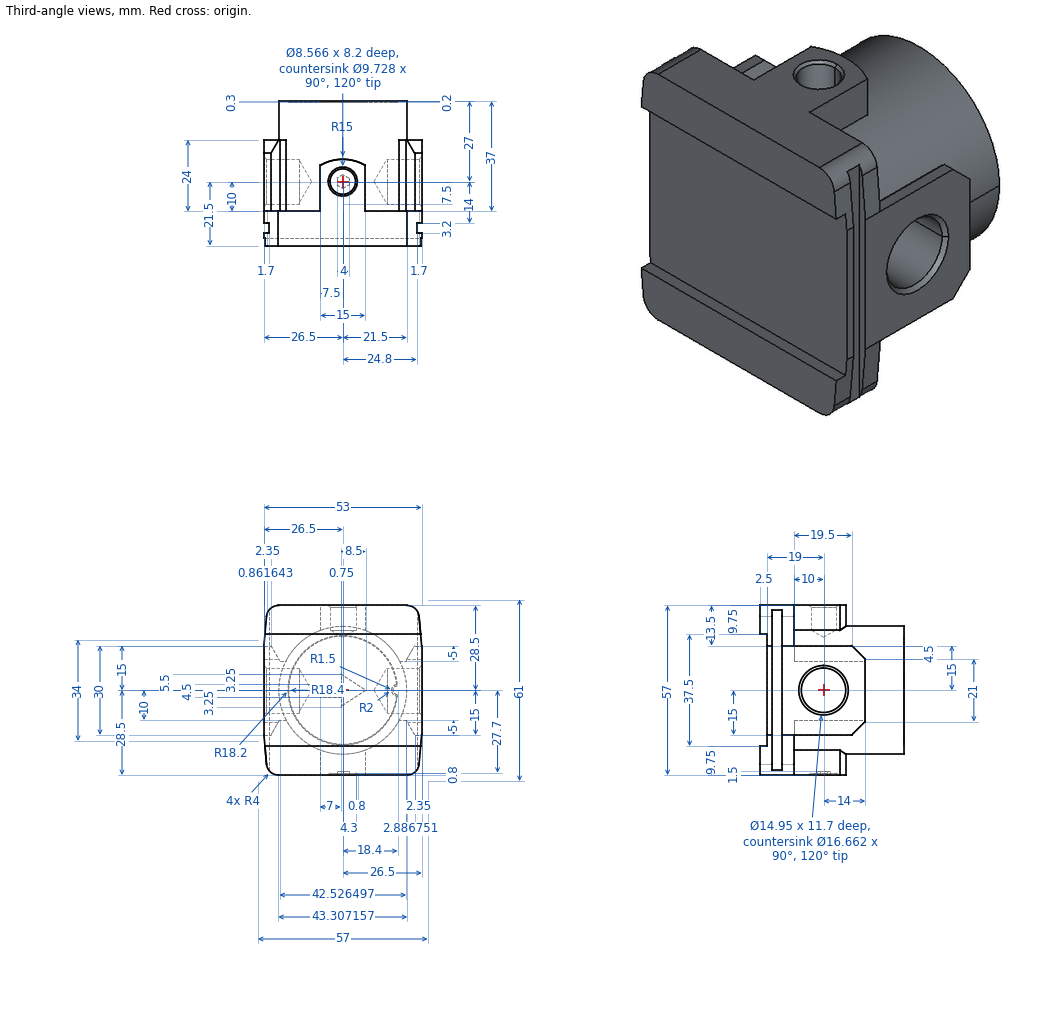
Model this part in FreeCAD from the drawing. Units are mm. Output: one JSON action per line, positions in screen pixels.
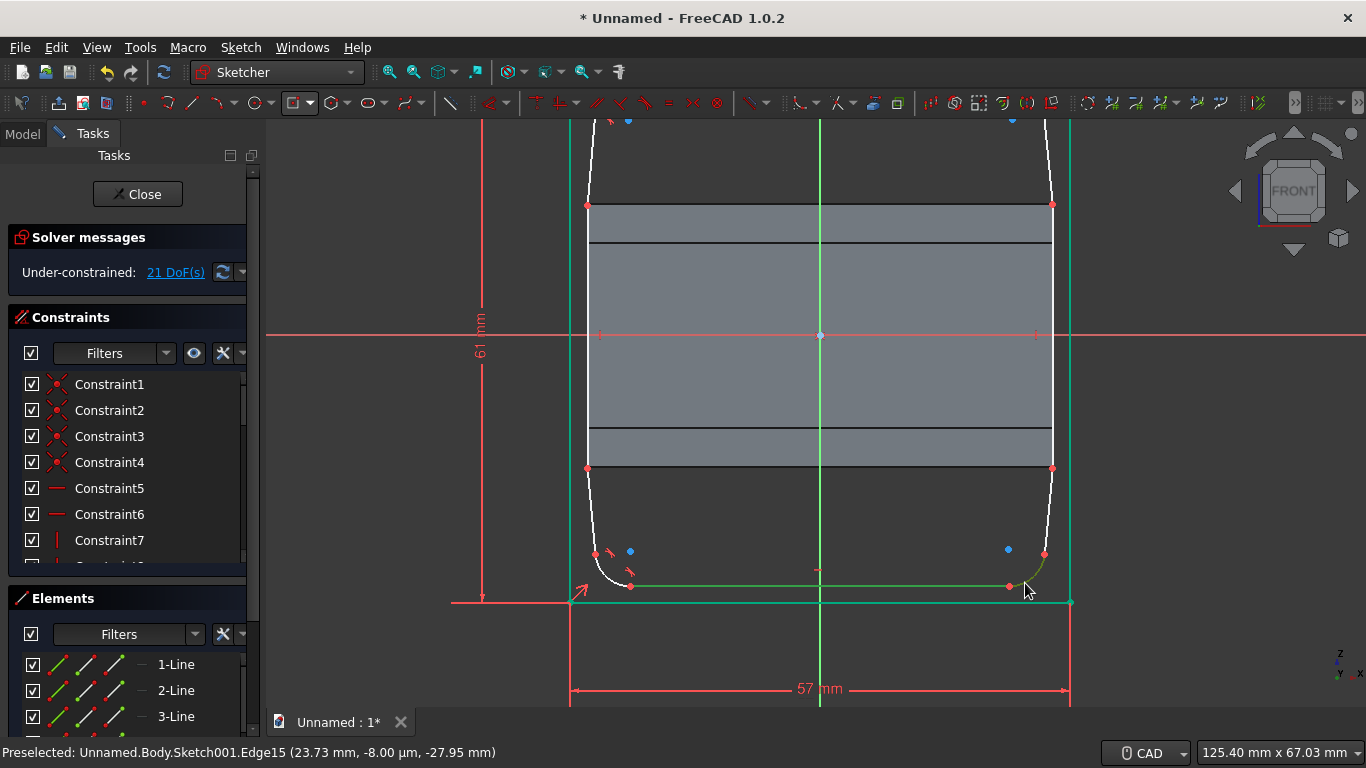
{"action": "key", "text": "t"}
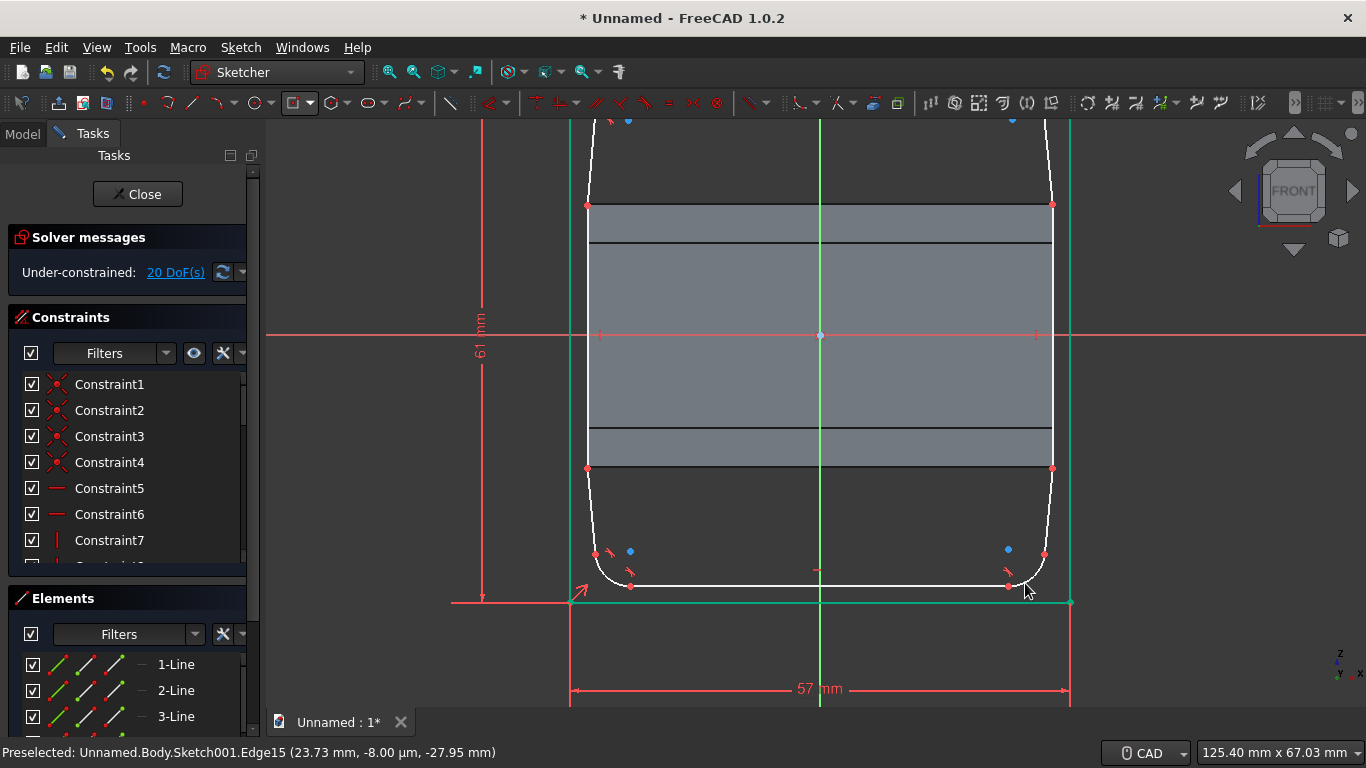
{"action": "left_click", "coordinate": [1047, 529]}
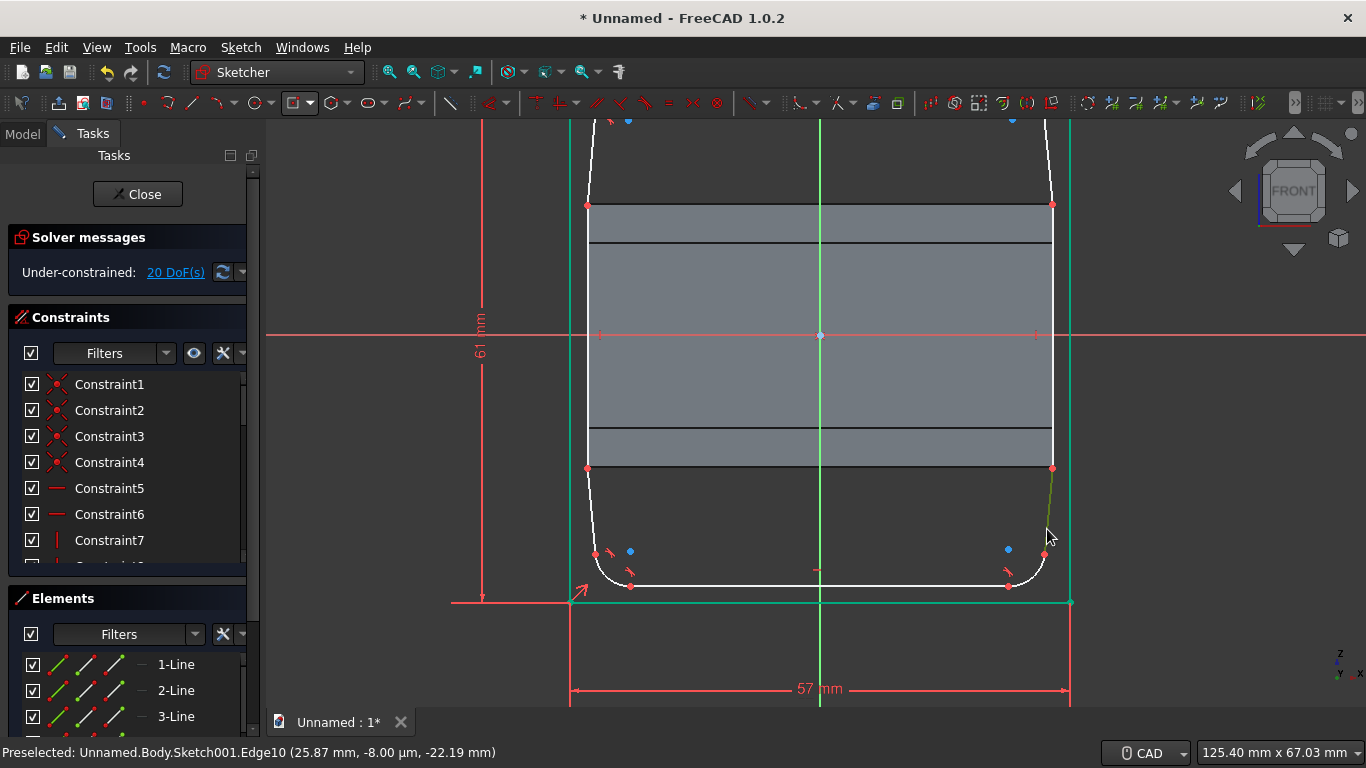
{"action": "left_click", "coordinate": [1024, 583]}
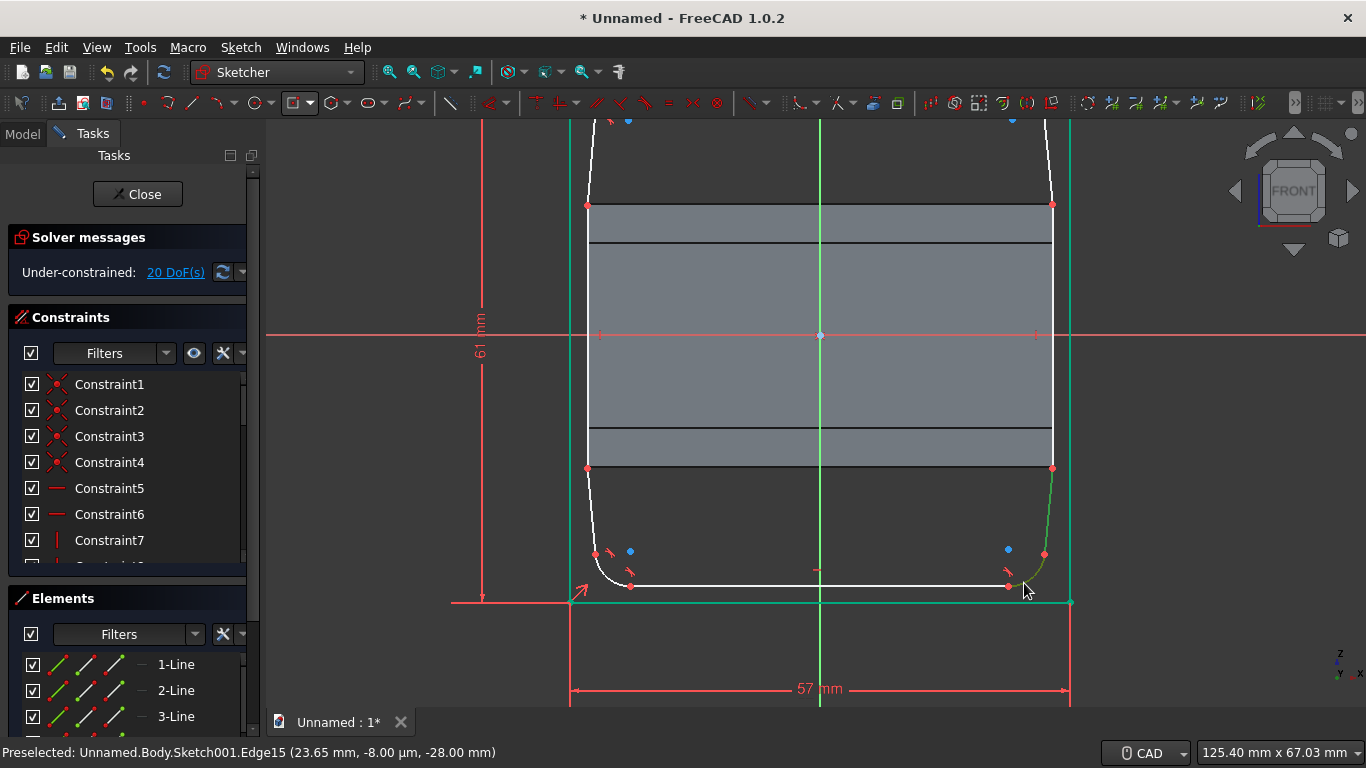
{"action": "key", "text": "t"}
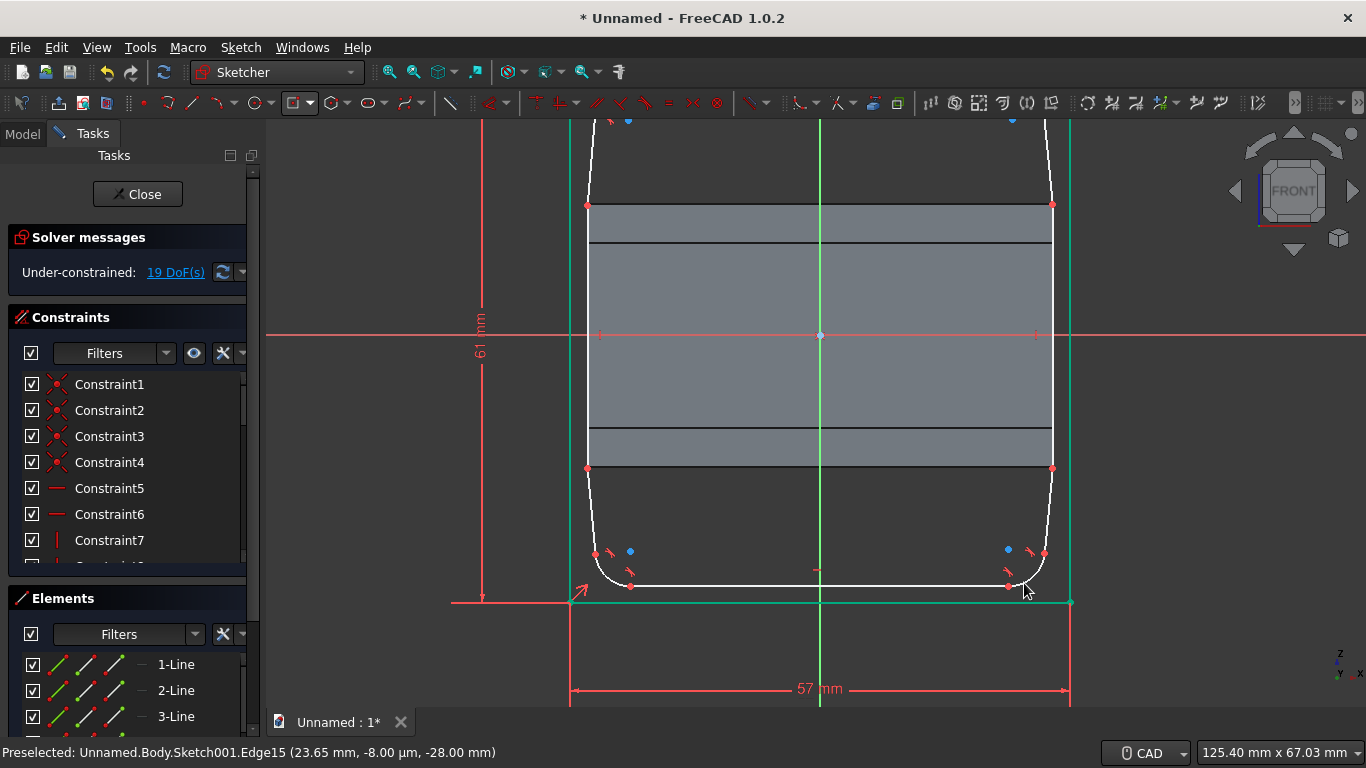
{"action": "left_click", "coordinate": [1050, 179]}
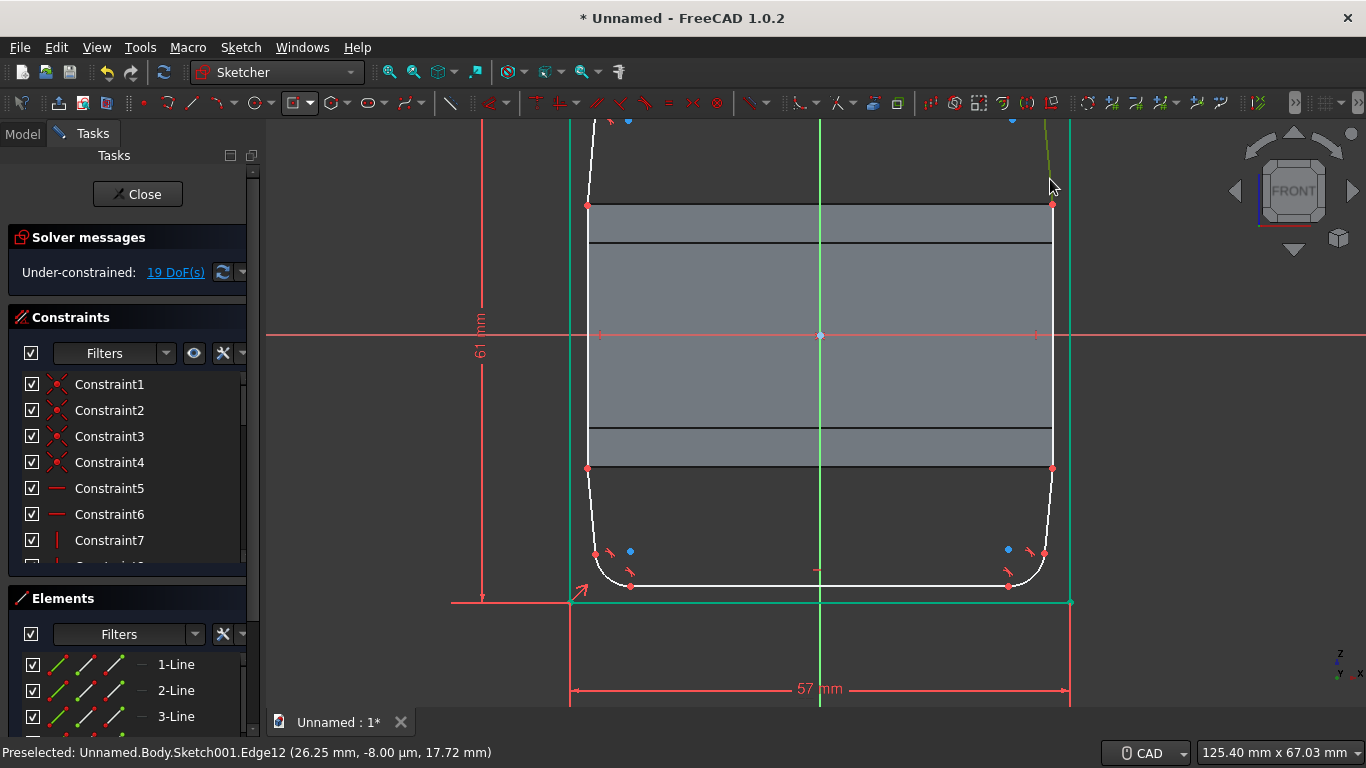
{"action": "scroll", "coordinate": [600, 571], "scroll_direction": "down", "scroll_amount": 2}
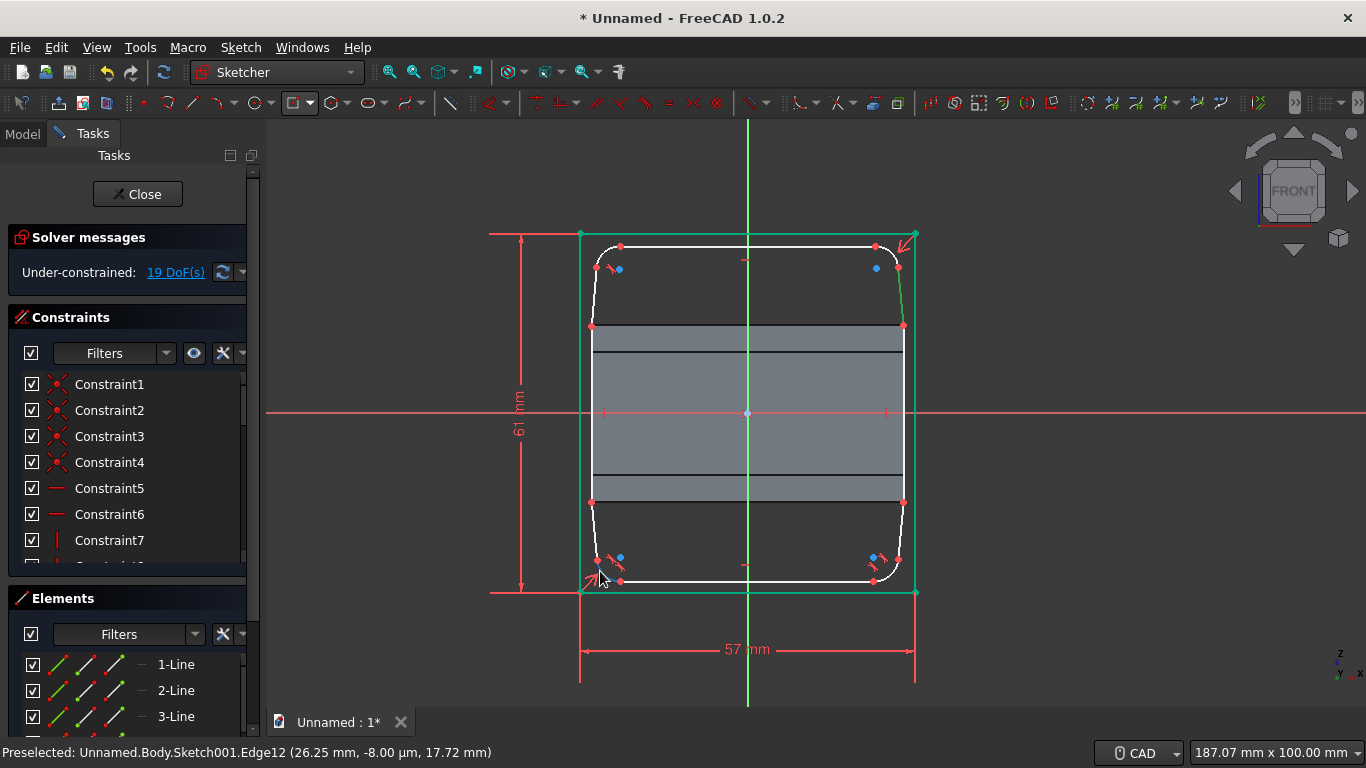
{"action": "scroll", "coordinate": [895, 258], "scroll_direction": "up", "scroll_amount": 2}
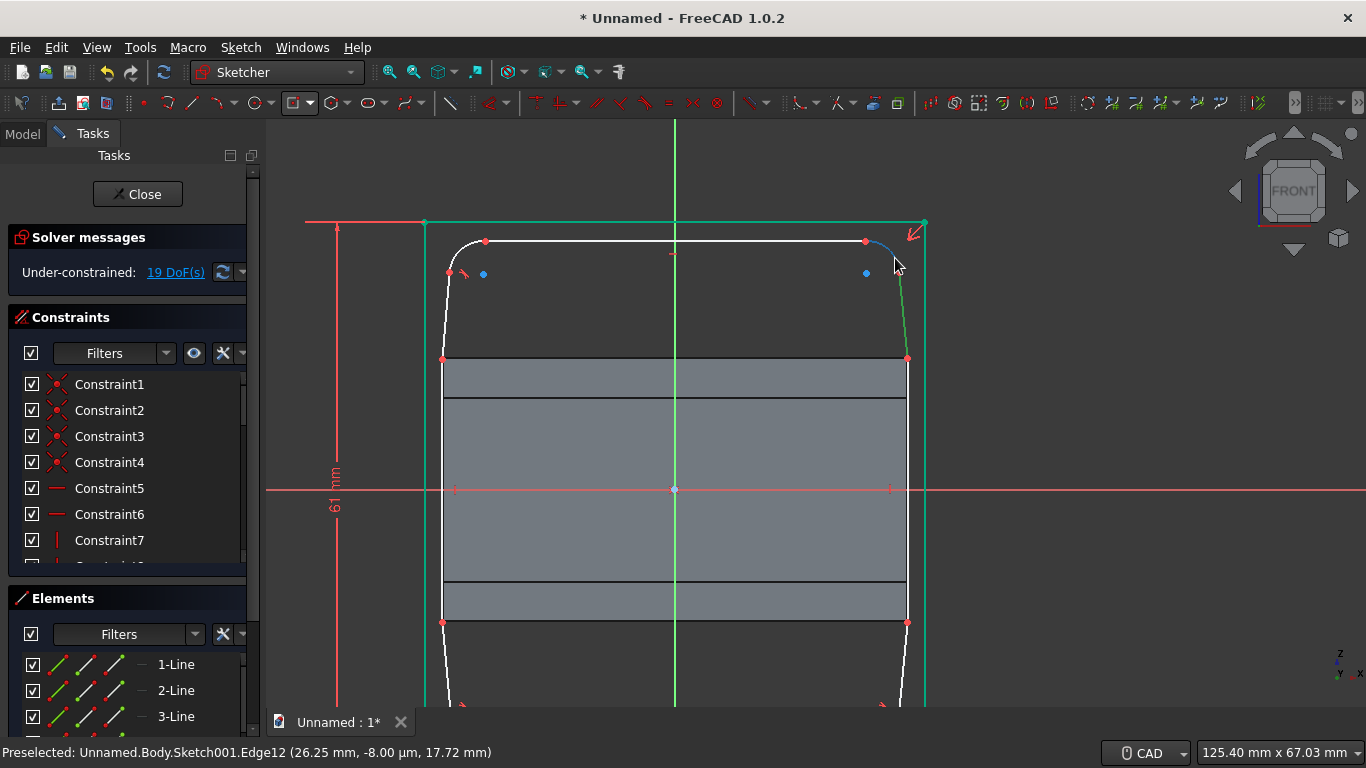
{"action": "left_click", "coordinate": [895, 258]}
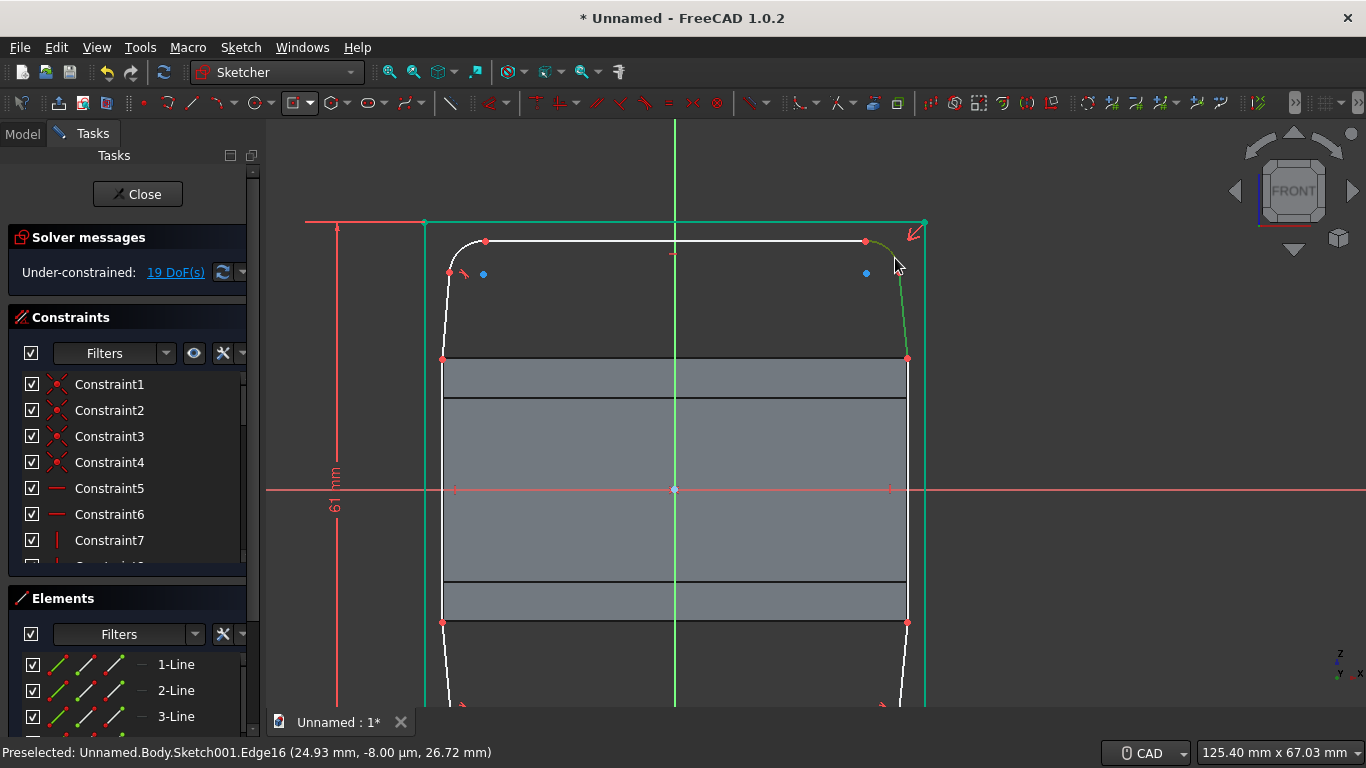
{"action": "key", "text": "t"}